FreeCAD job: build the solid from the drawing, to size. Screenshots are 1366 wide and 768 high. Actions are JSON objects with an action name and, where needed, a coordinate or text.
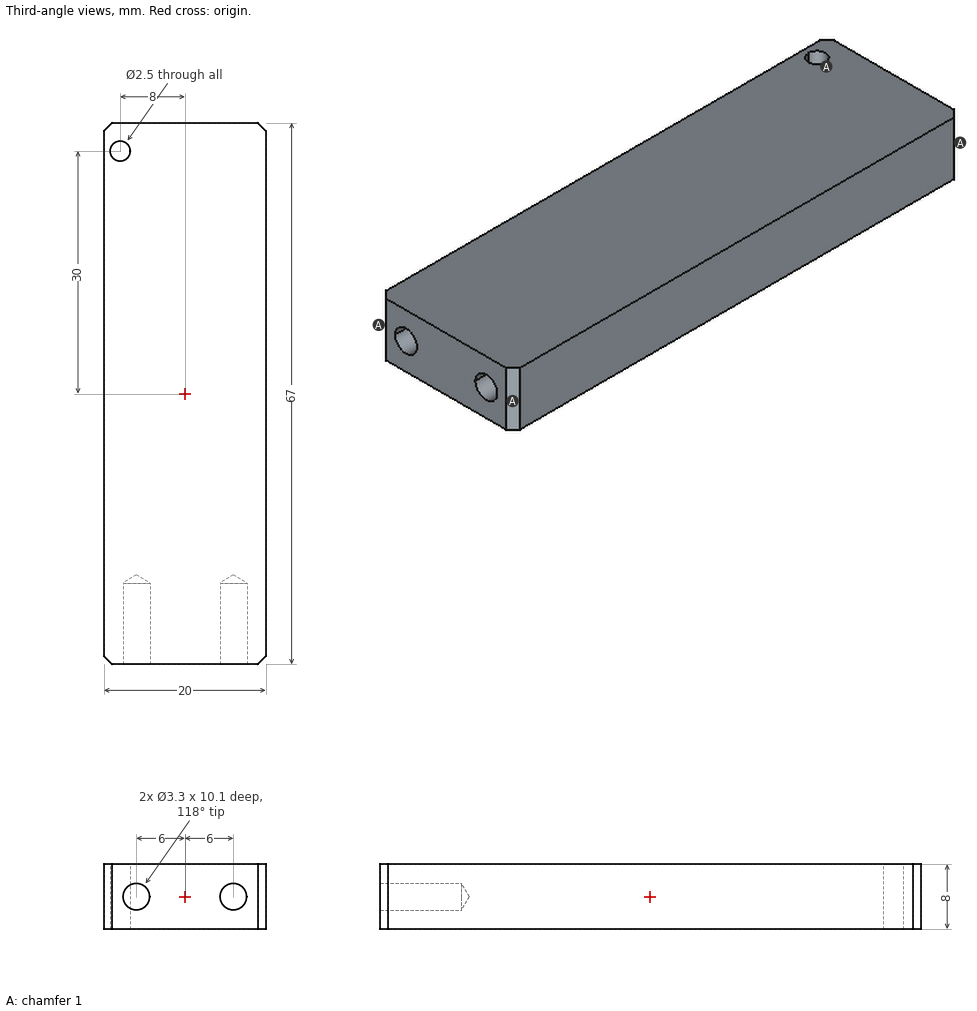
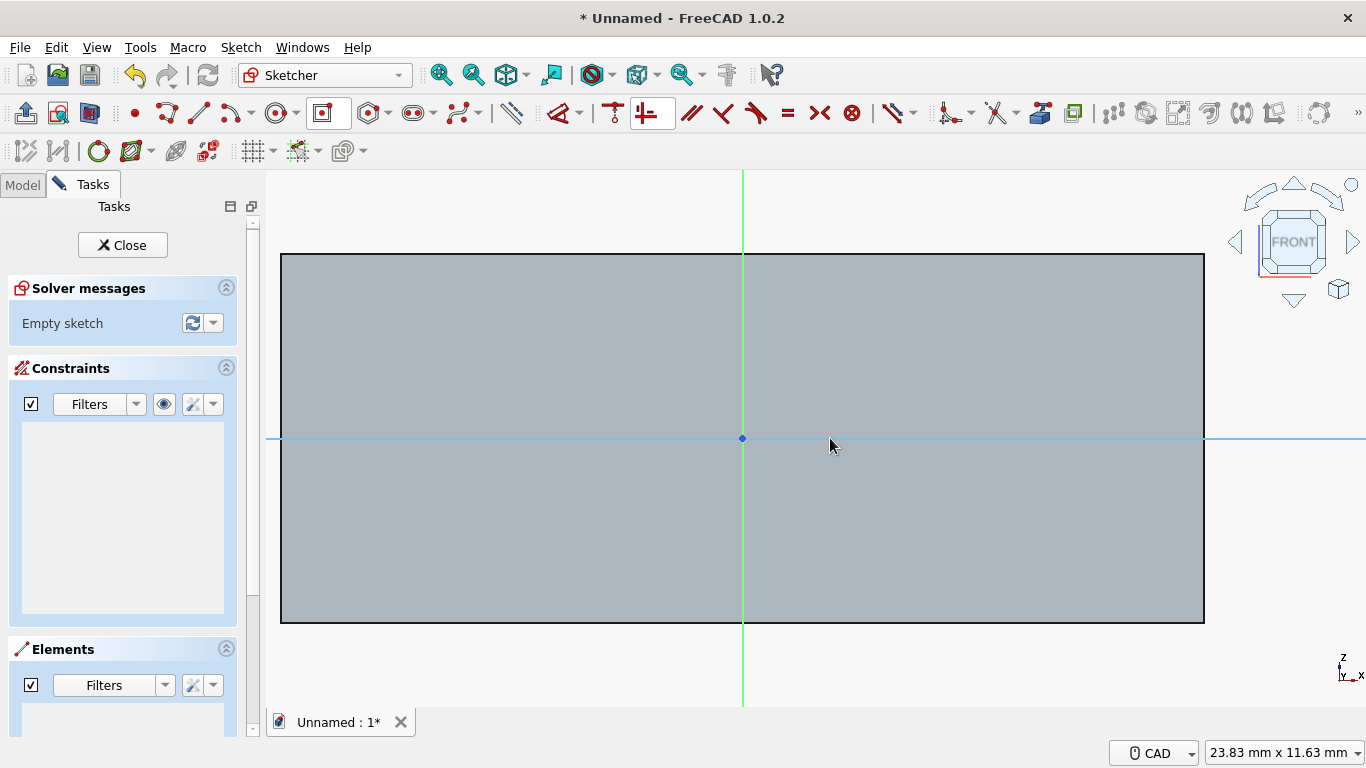
{"action": "key", "text": "g c"}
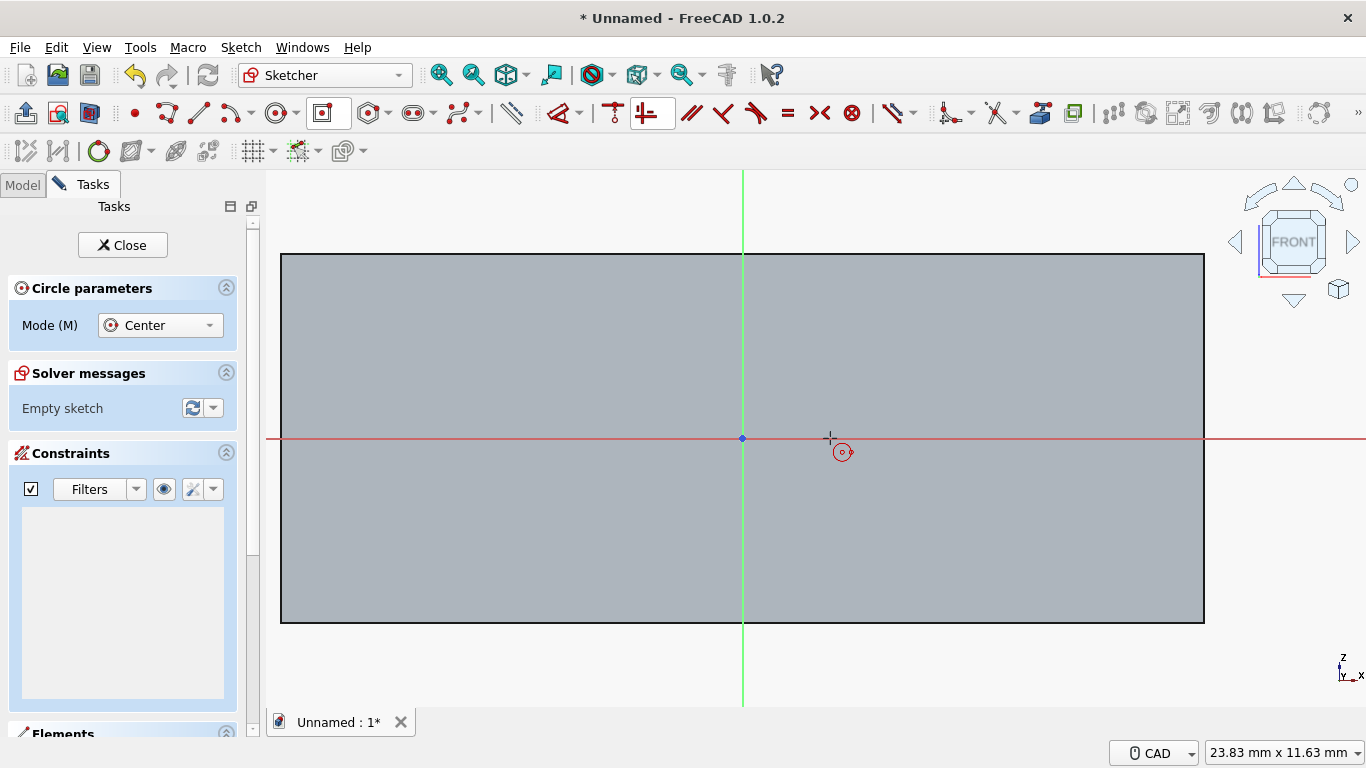
{"action": "left_click", "coordinate": [466, 438]}
{"action": "mouse_move", "coordinate": [520, 385]}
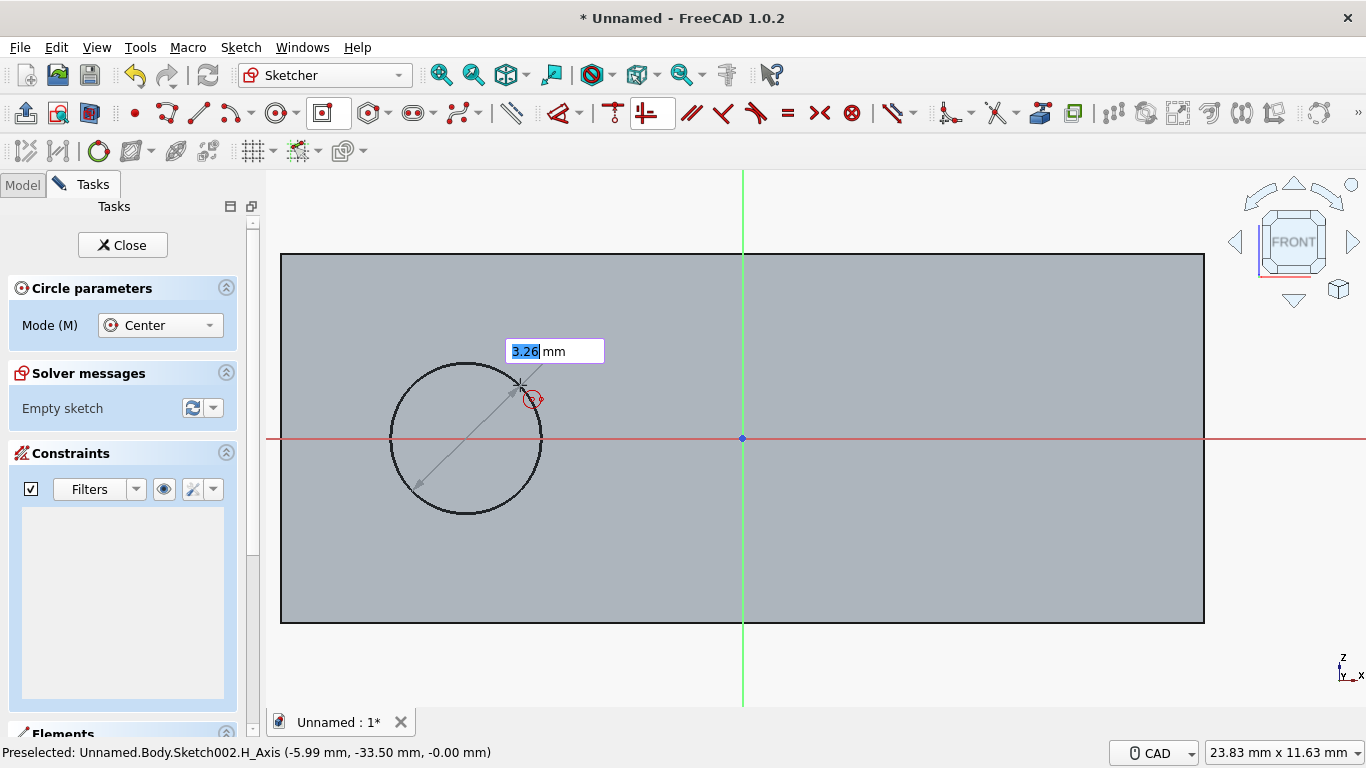
{"action": "type", "text": "3.3"}
{"action": "key", "text": "Return"}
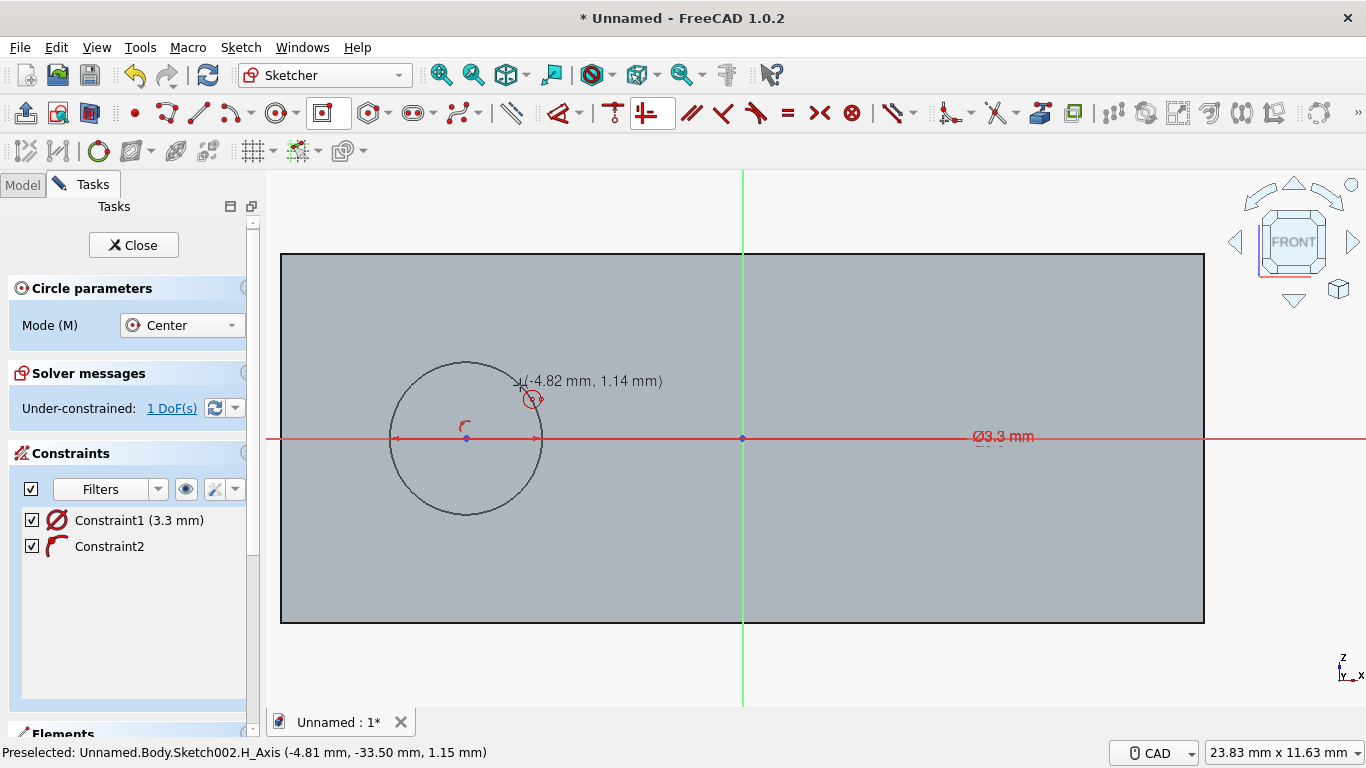
{"action": "left_click", "coordinate": [1020, 438]}
{"action": "mouse_move", "coordinate": [1074, 385]}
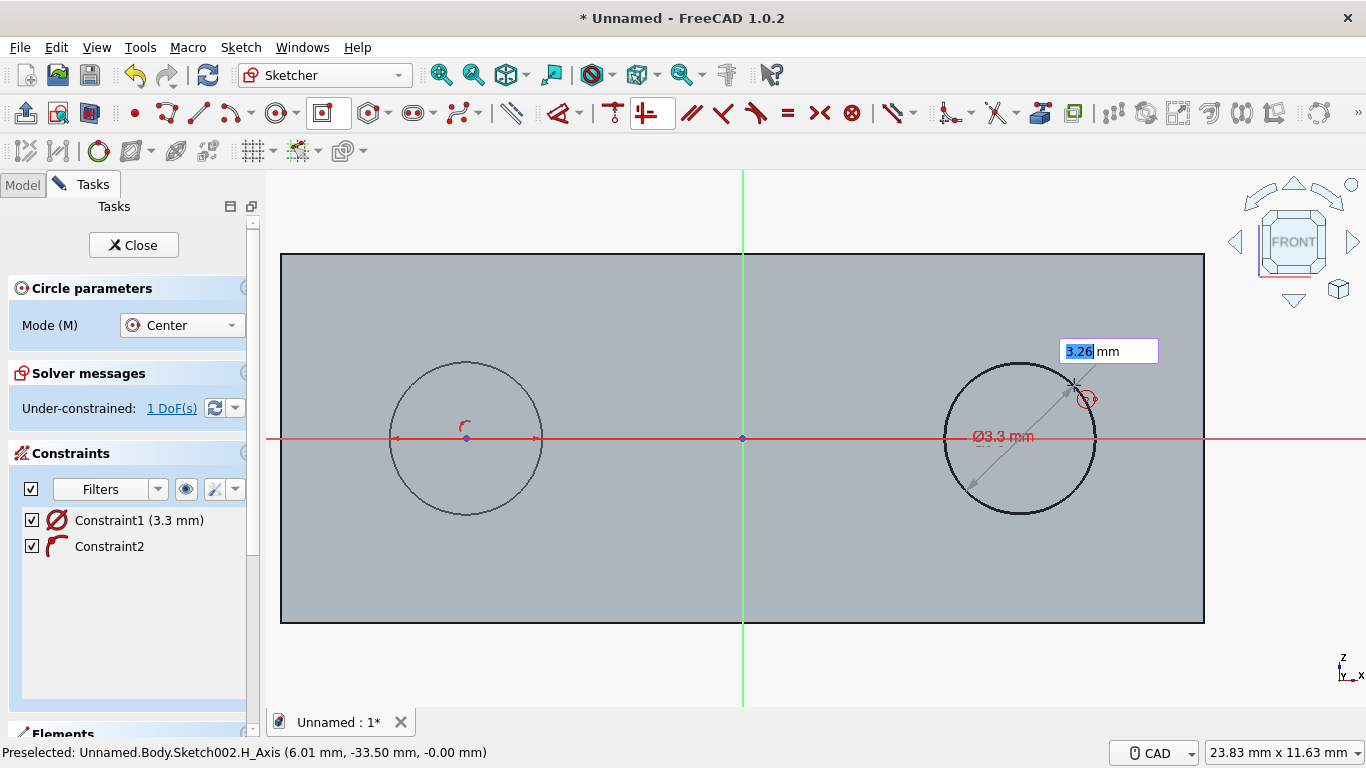
{"action": "type", "text": "3.3"}
{"action": "key", "text": "Return"}
{"action": "key", "text": "Escape"}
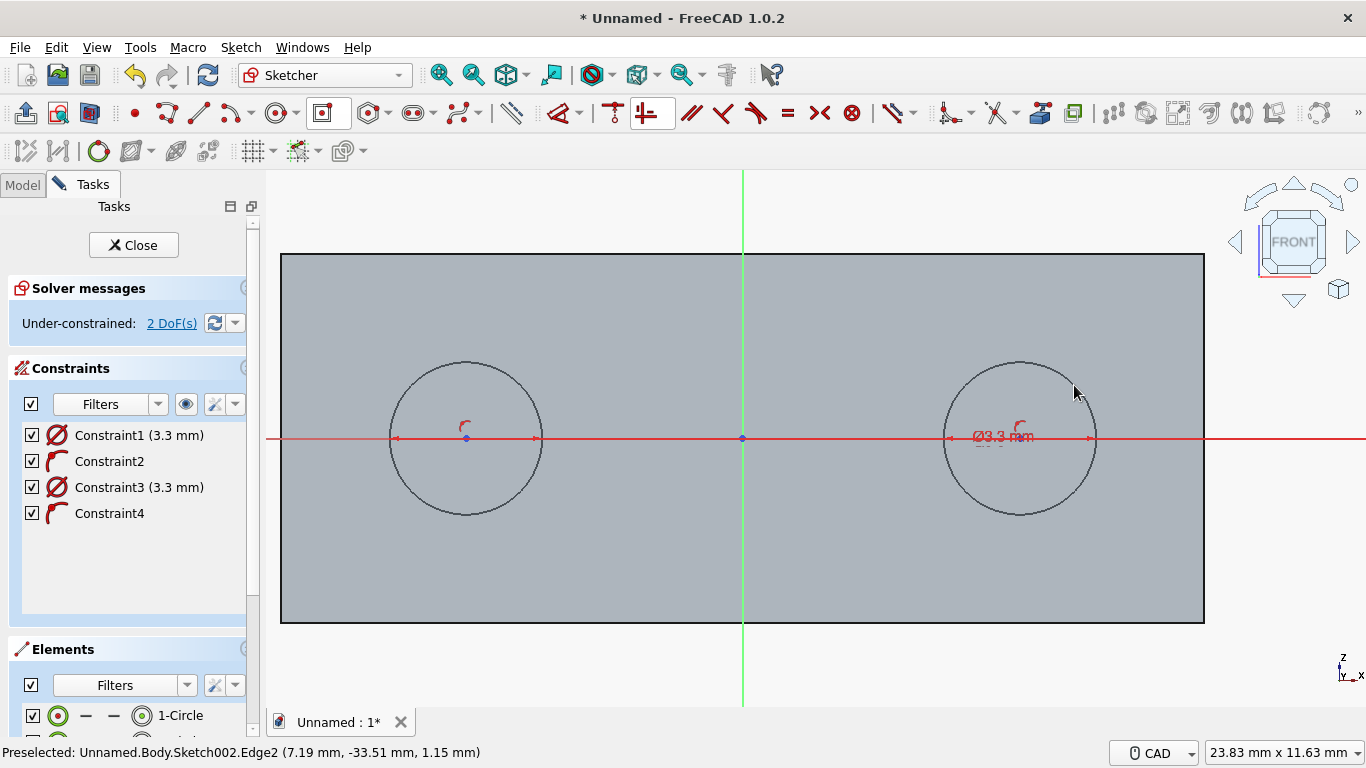
{"action": "key", "text": "d"}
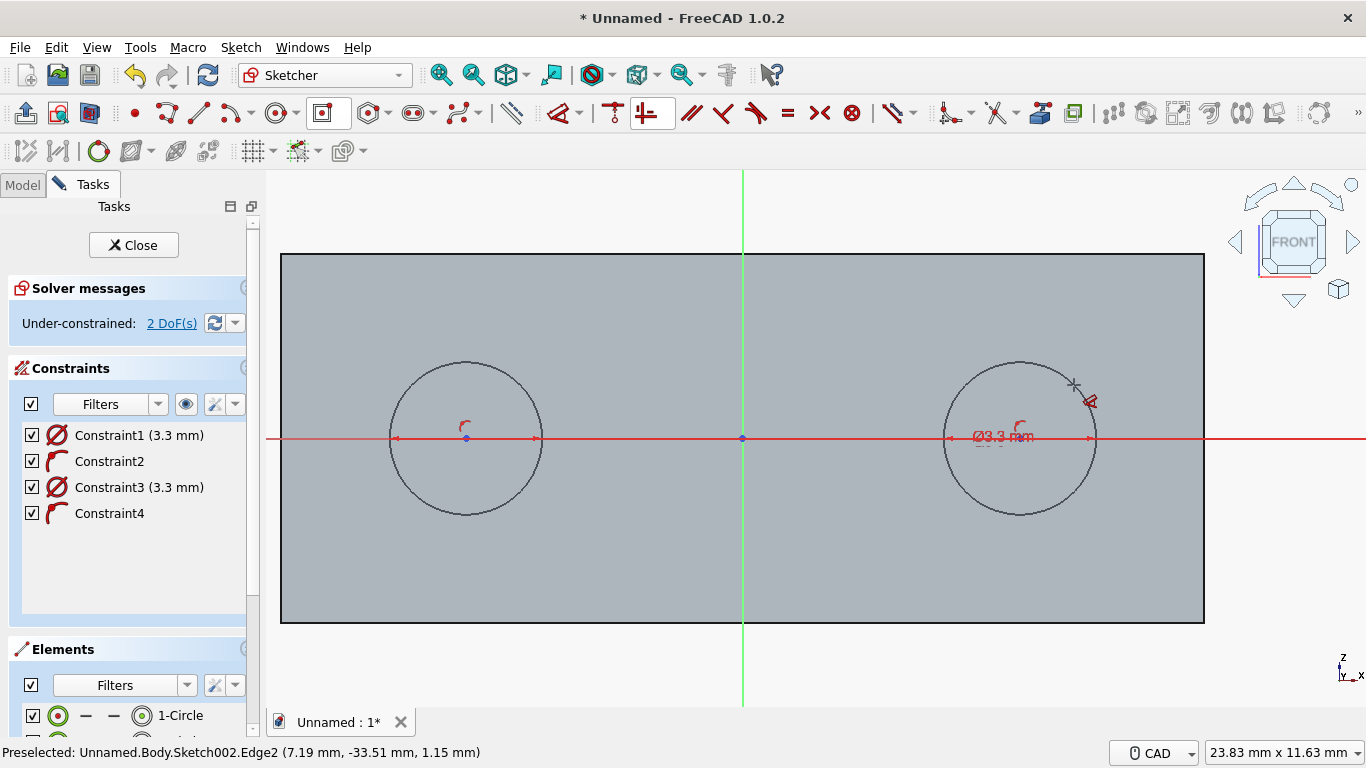
{"action": "left_click", "coordinate": [466, 438]}
{"action": "left_click", "coordinate": [604, 472]}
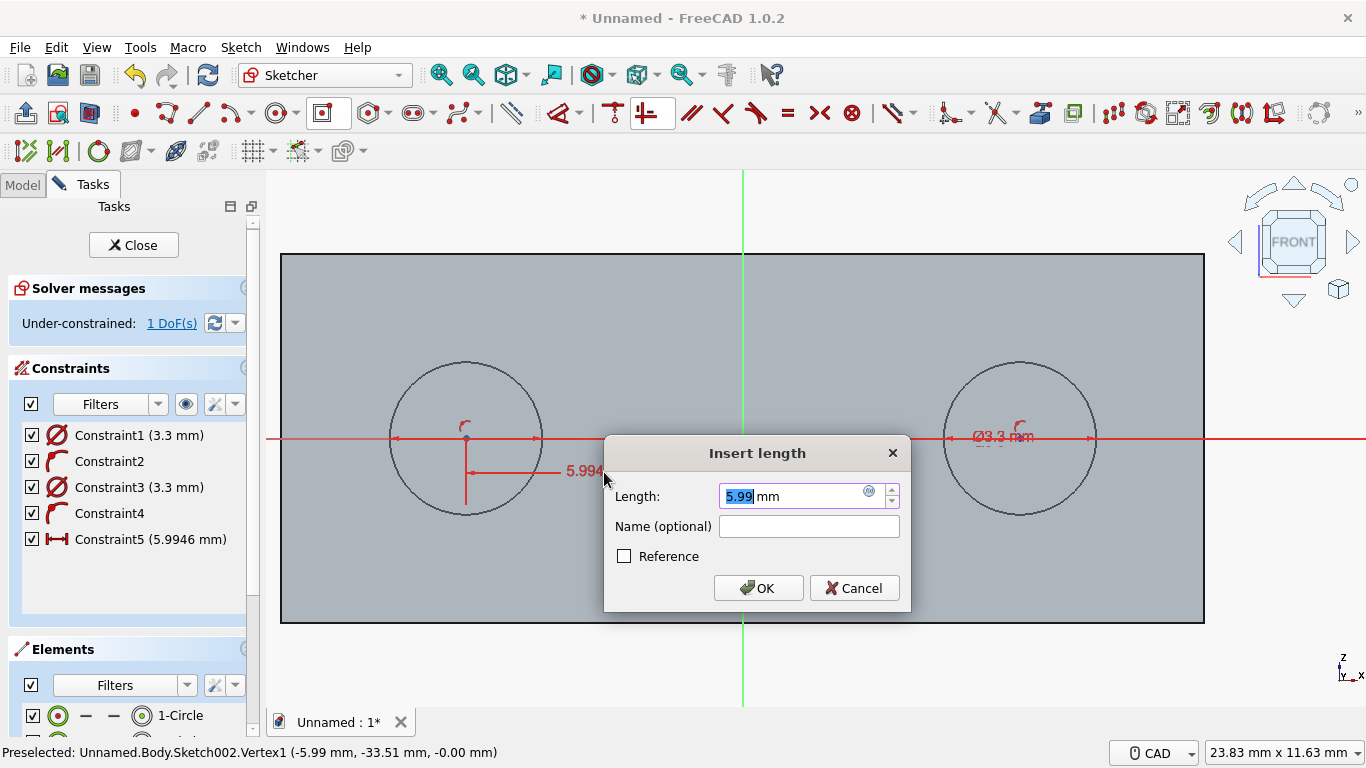
{"action": "type", "text": "6"}
{"action": "key", "text": "Return"}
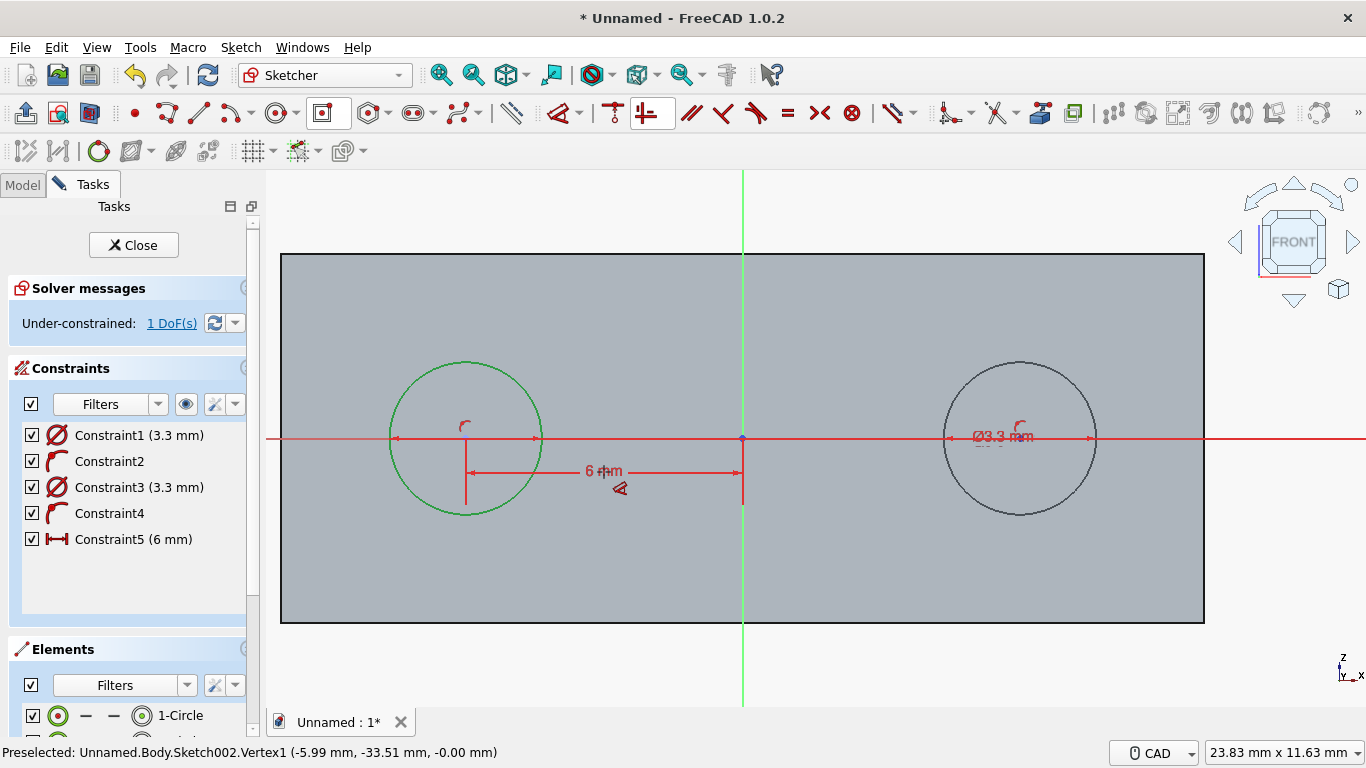
{"action": "left_click", "coordinate": [1020, 438]}
{"action": "left_click", "coordinate": [881, 472]}